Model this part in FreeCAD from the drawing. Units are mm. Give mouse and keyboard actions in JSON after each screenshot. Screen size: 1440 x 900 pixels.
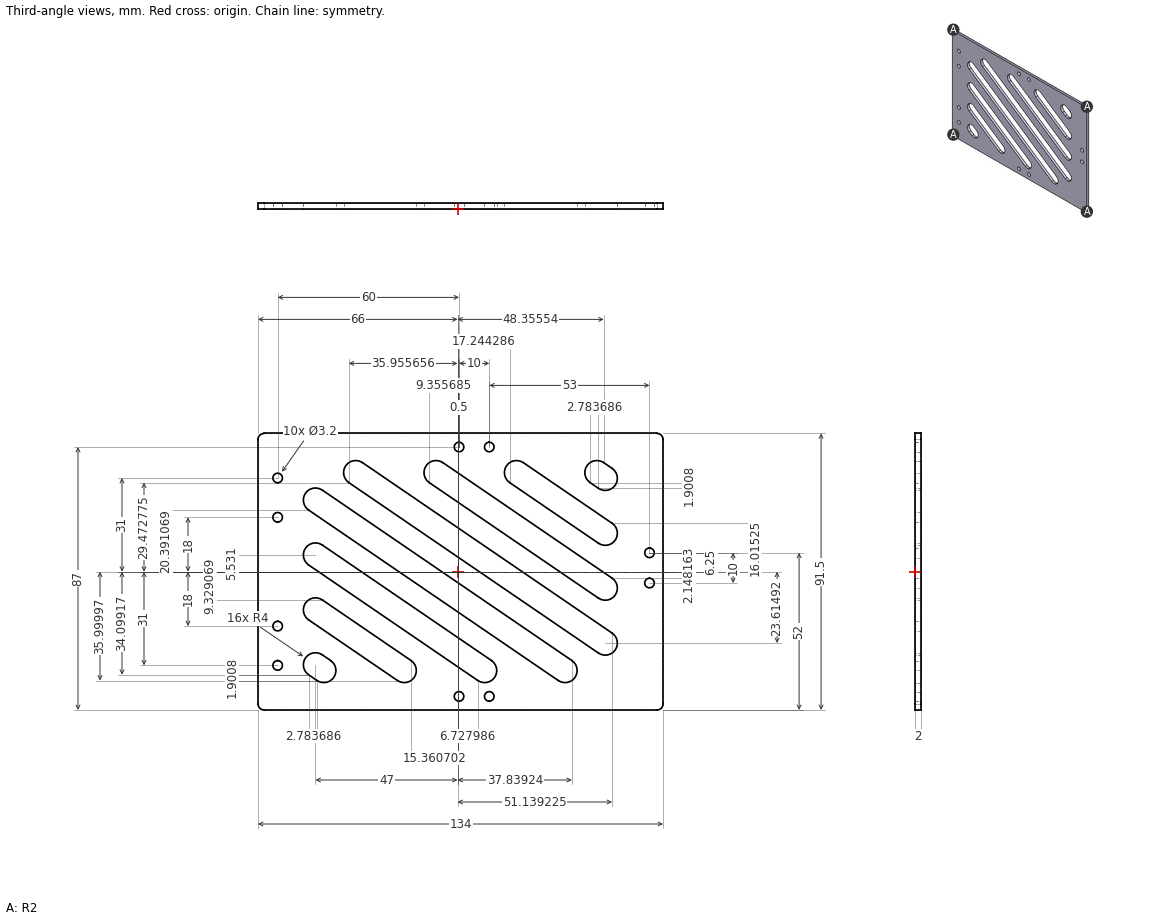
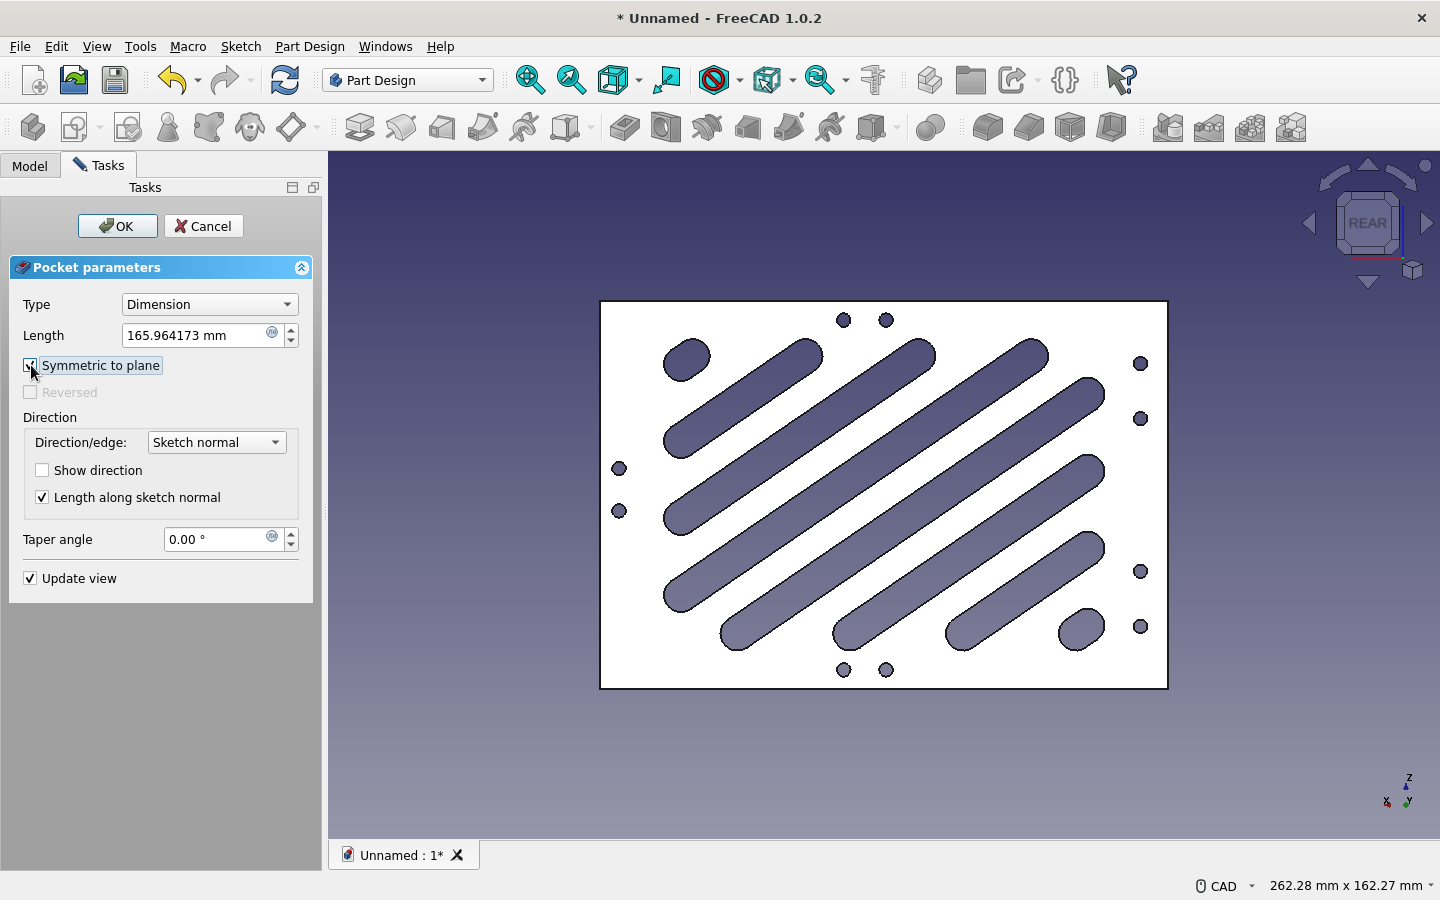
{"action": "left_click", "coordinate": [118, 226]}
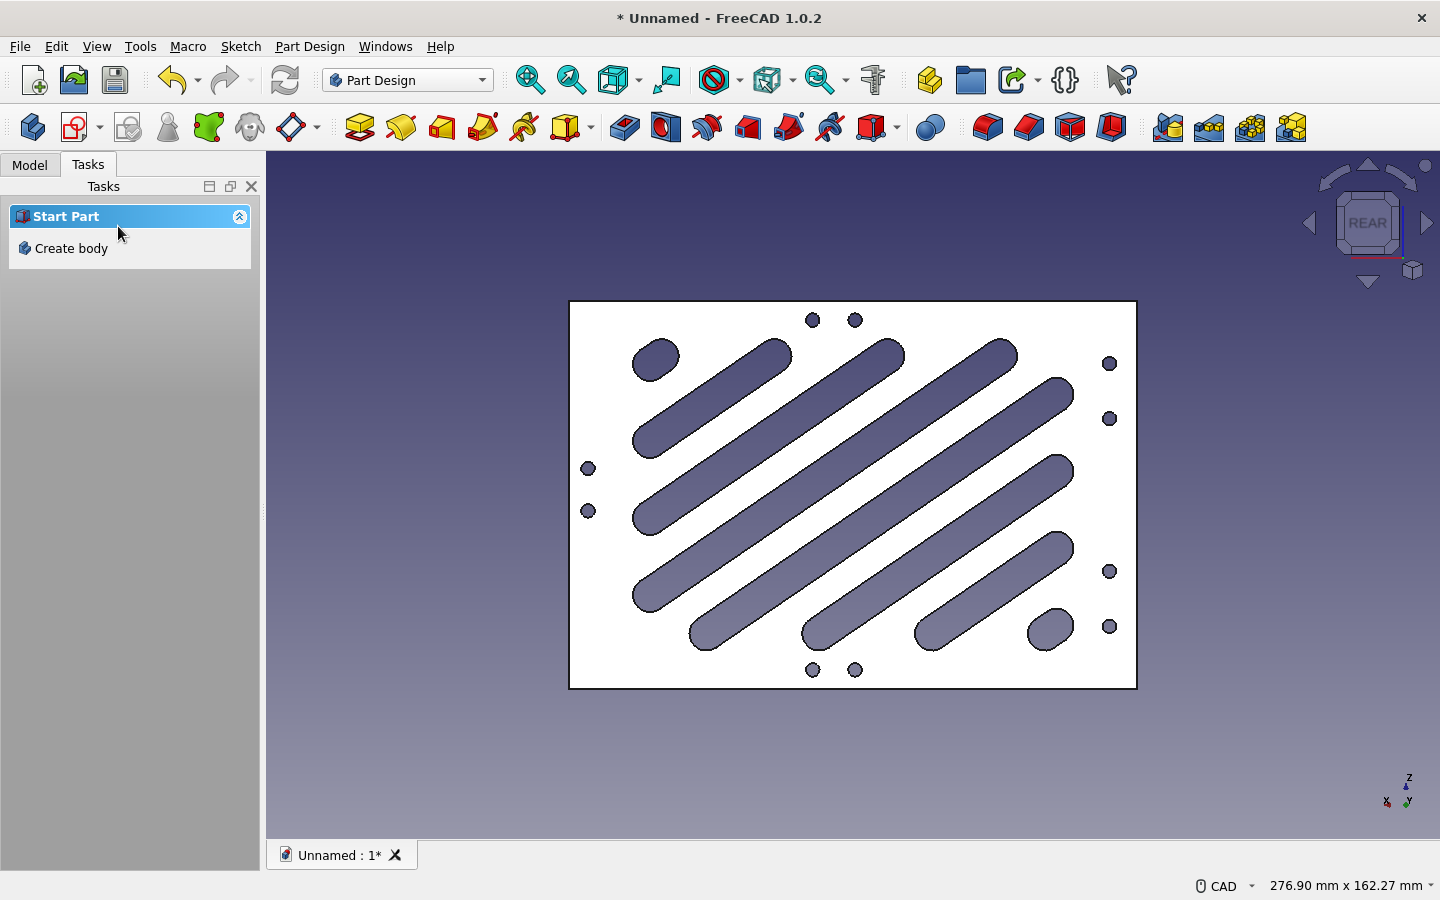
{"action": "scroll", "coordinate": [1137, 688], "scroll_direction": "up", "scroll_amount": 8}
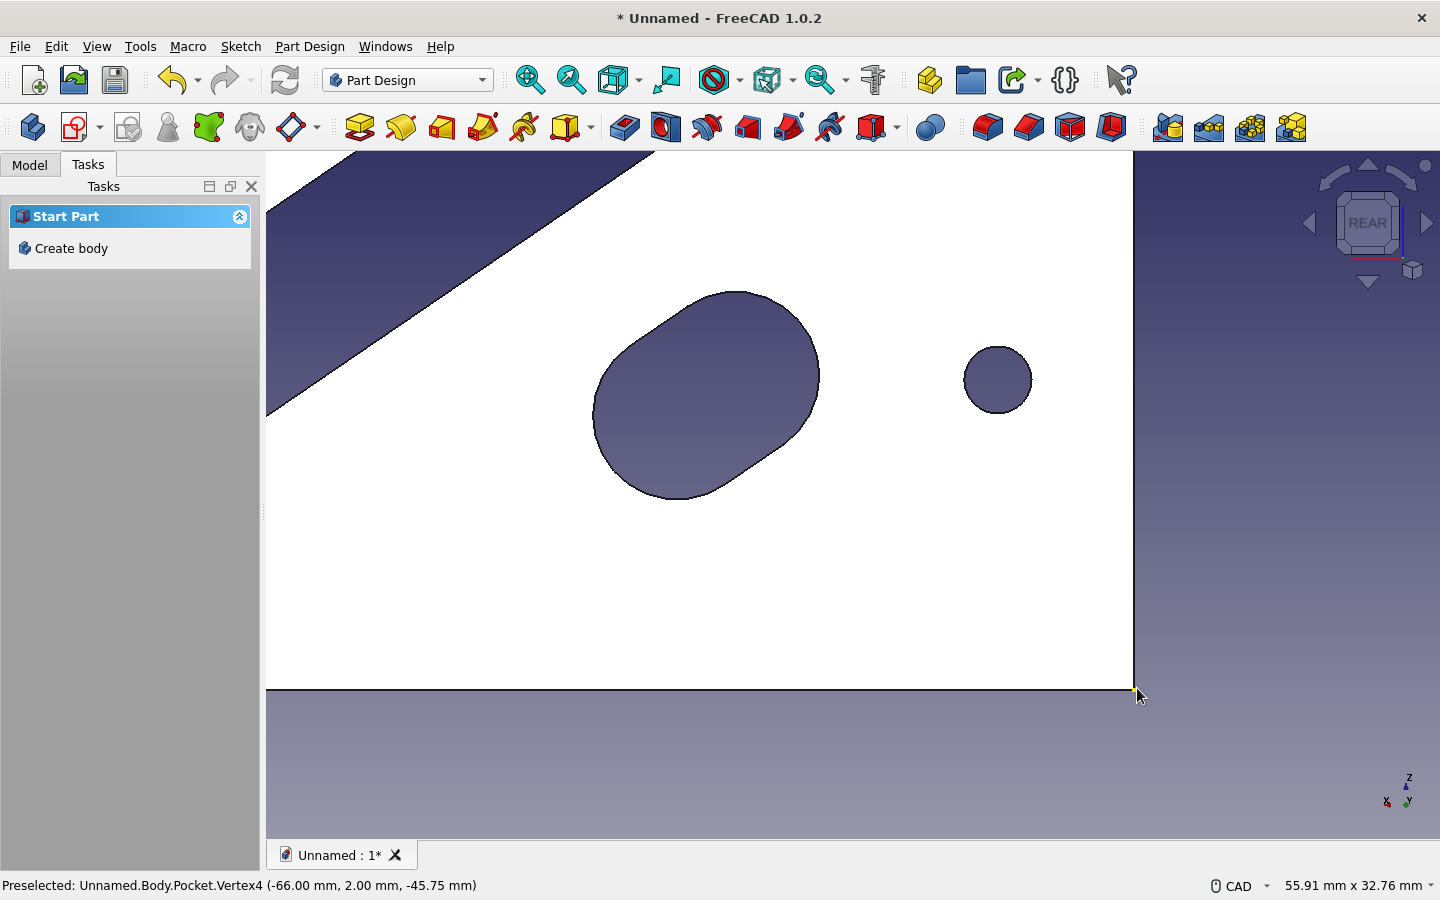
{"action": "left_click", "coordinate": [531, 80]}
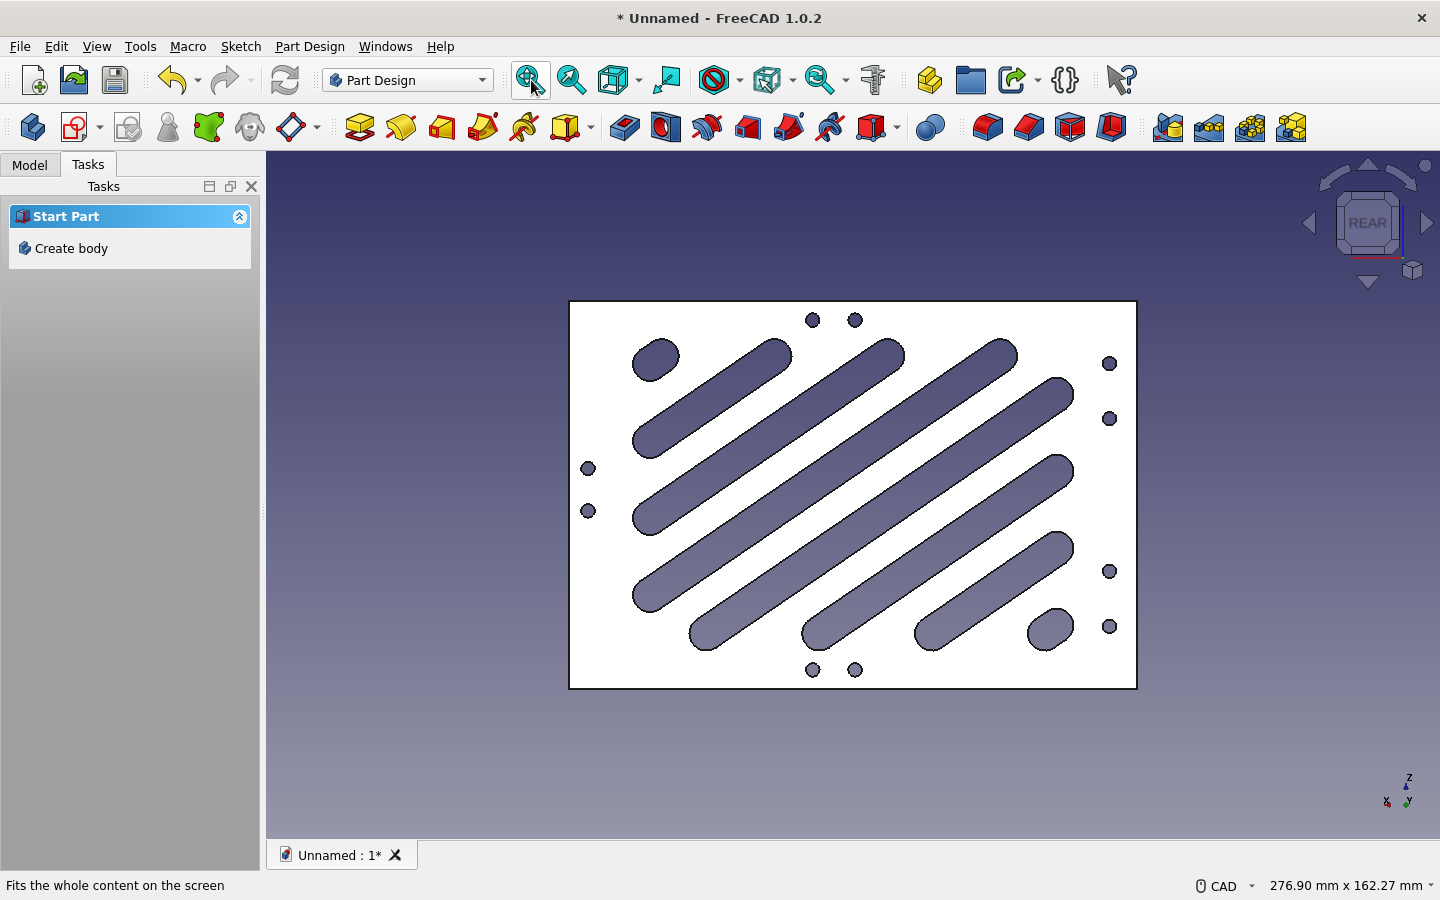
{"action": "key", "text": "0"}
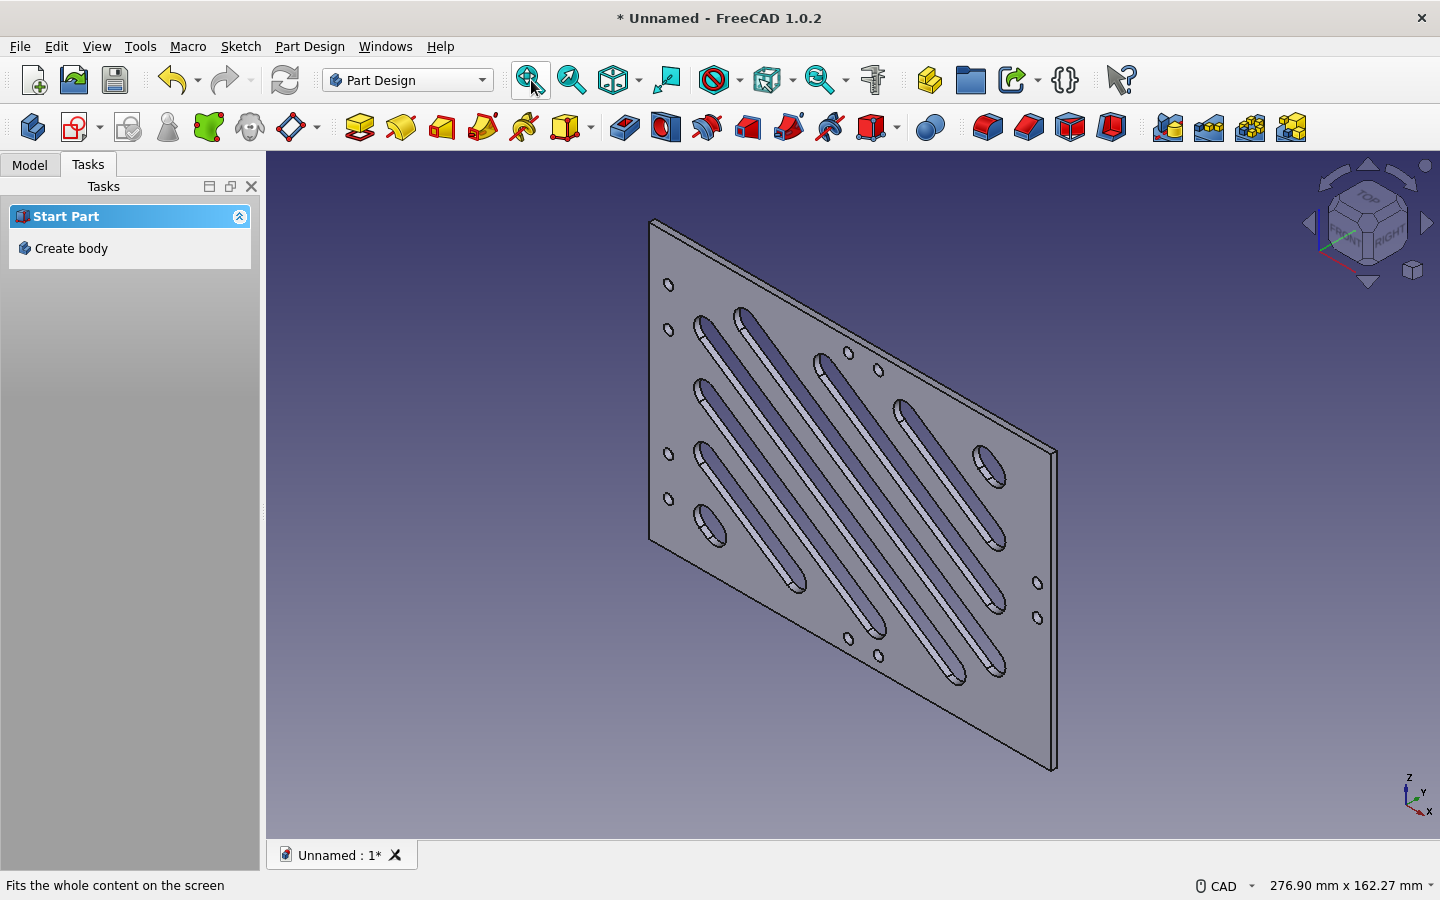
{"action": "scroll", "coordinate": [652, 536], "scroll_direction": "up", "scroll_amount": 8}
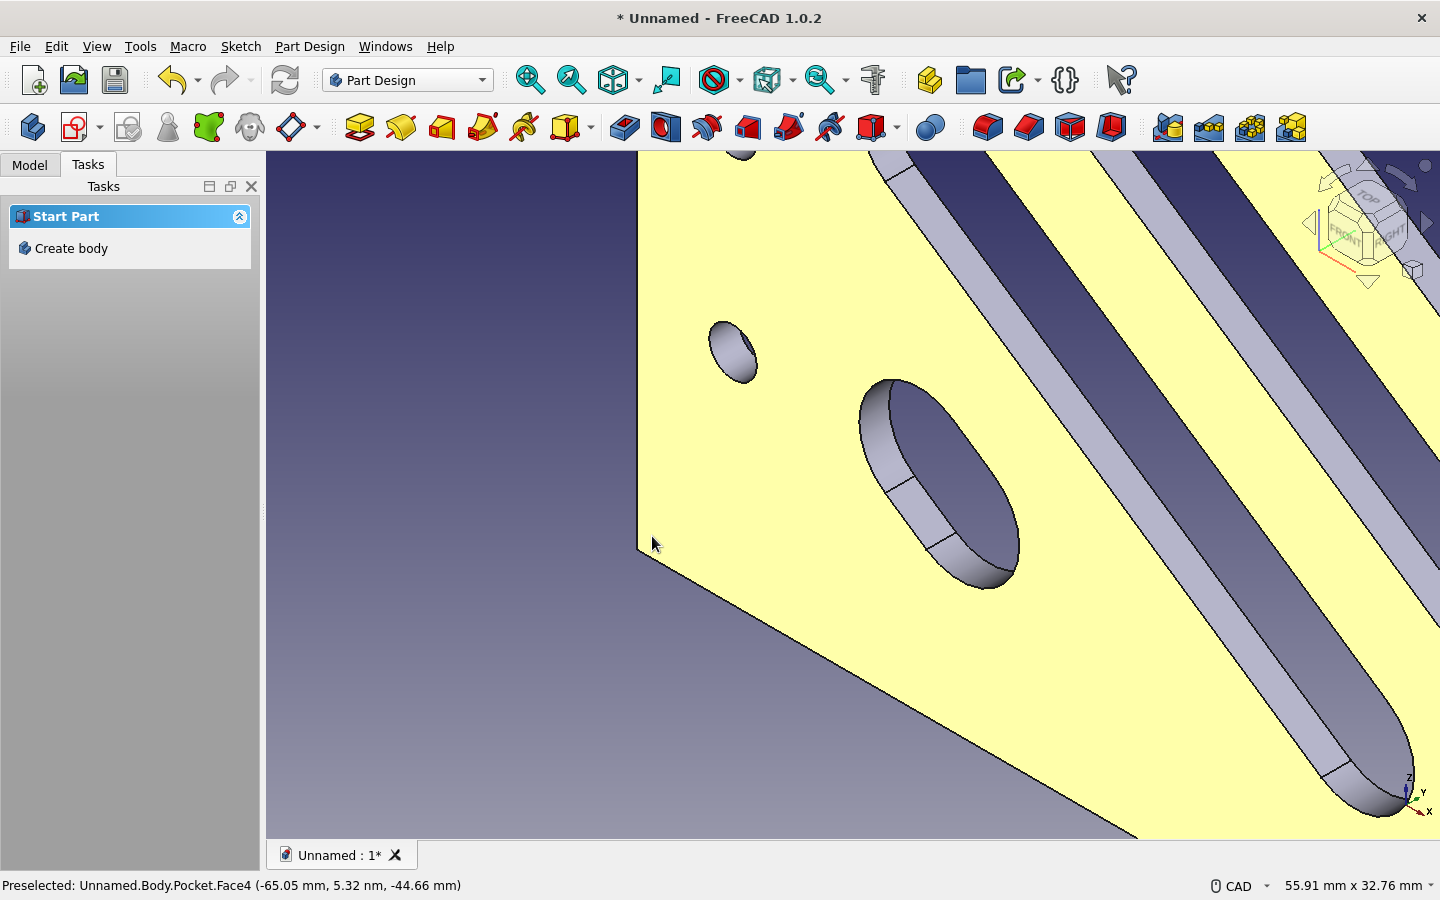
{"action": "left_click", "coordinate": [531, 80]}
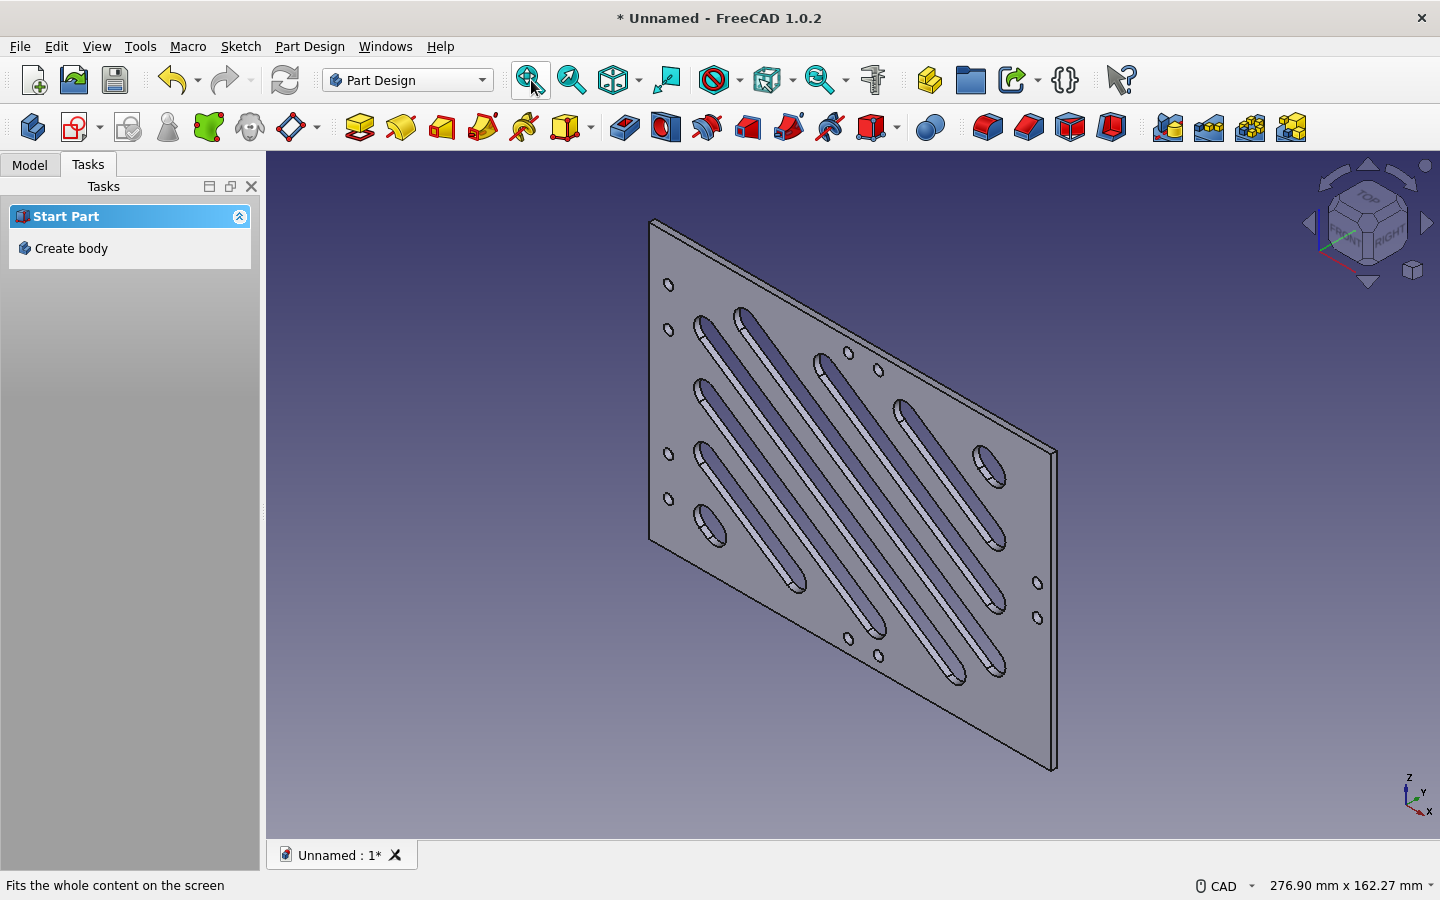
{"action": "key", "text": "2"}